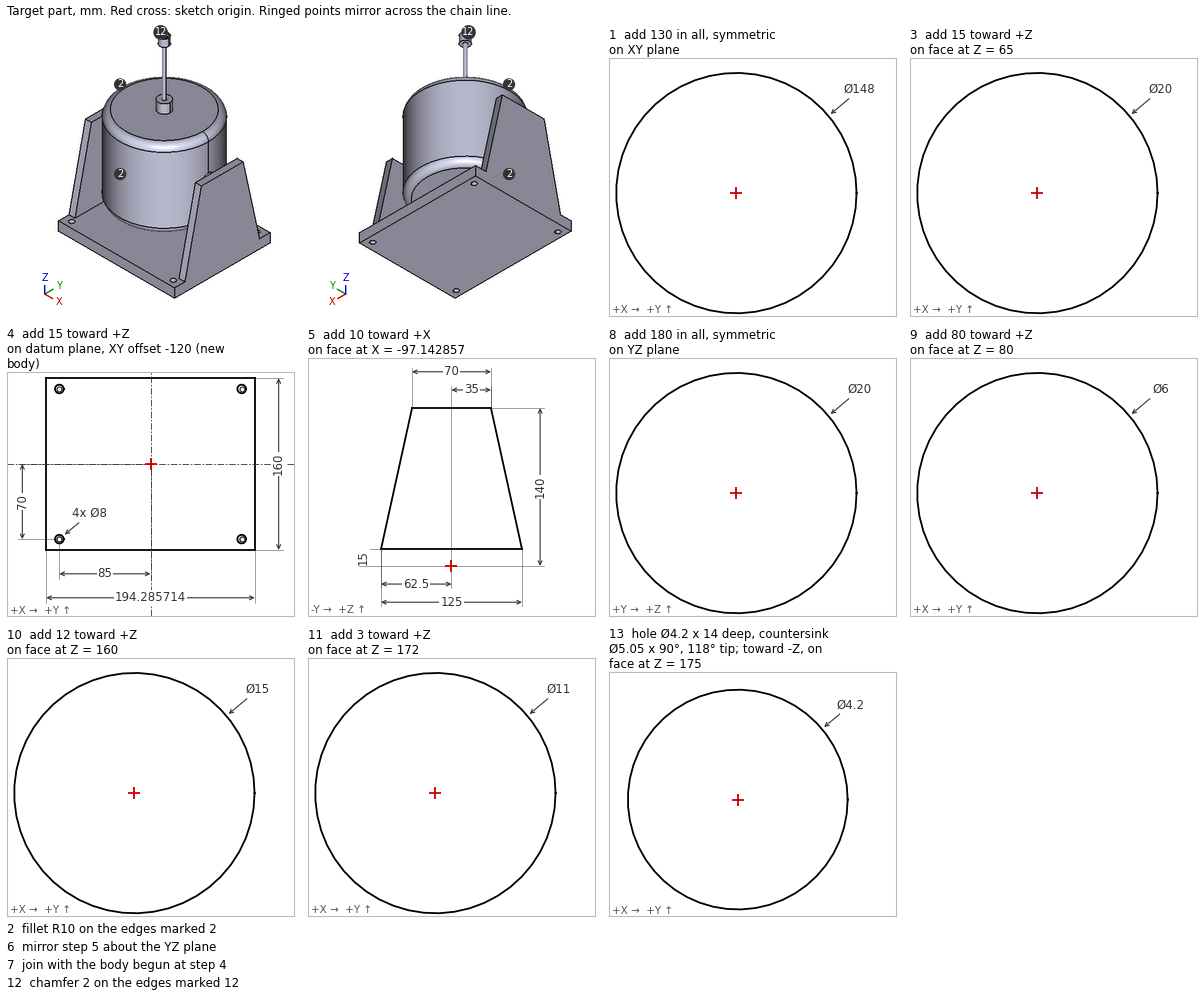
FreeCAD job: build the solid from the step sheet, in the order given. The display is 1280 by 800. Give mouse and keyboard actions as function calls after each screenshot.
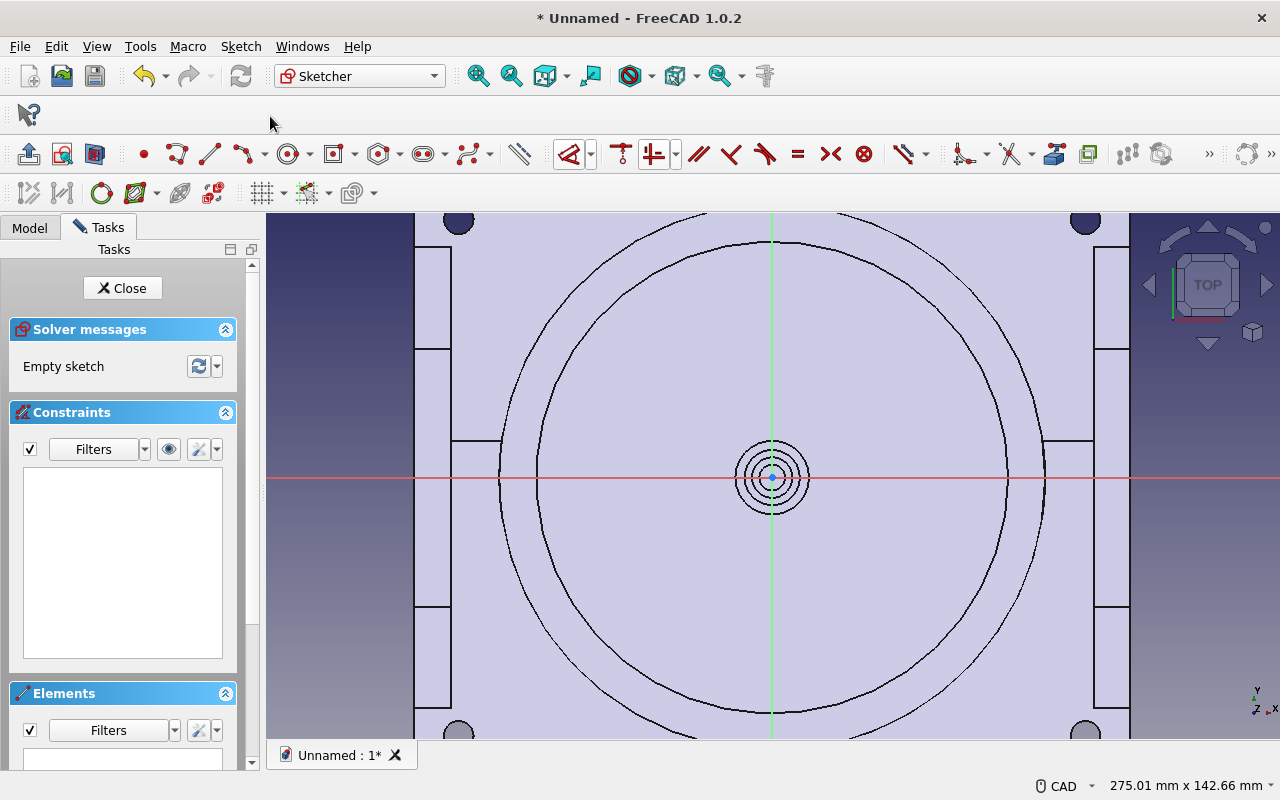
scroll(776, 478, up, 15)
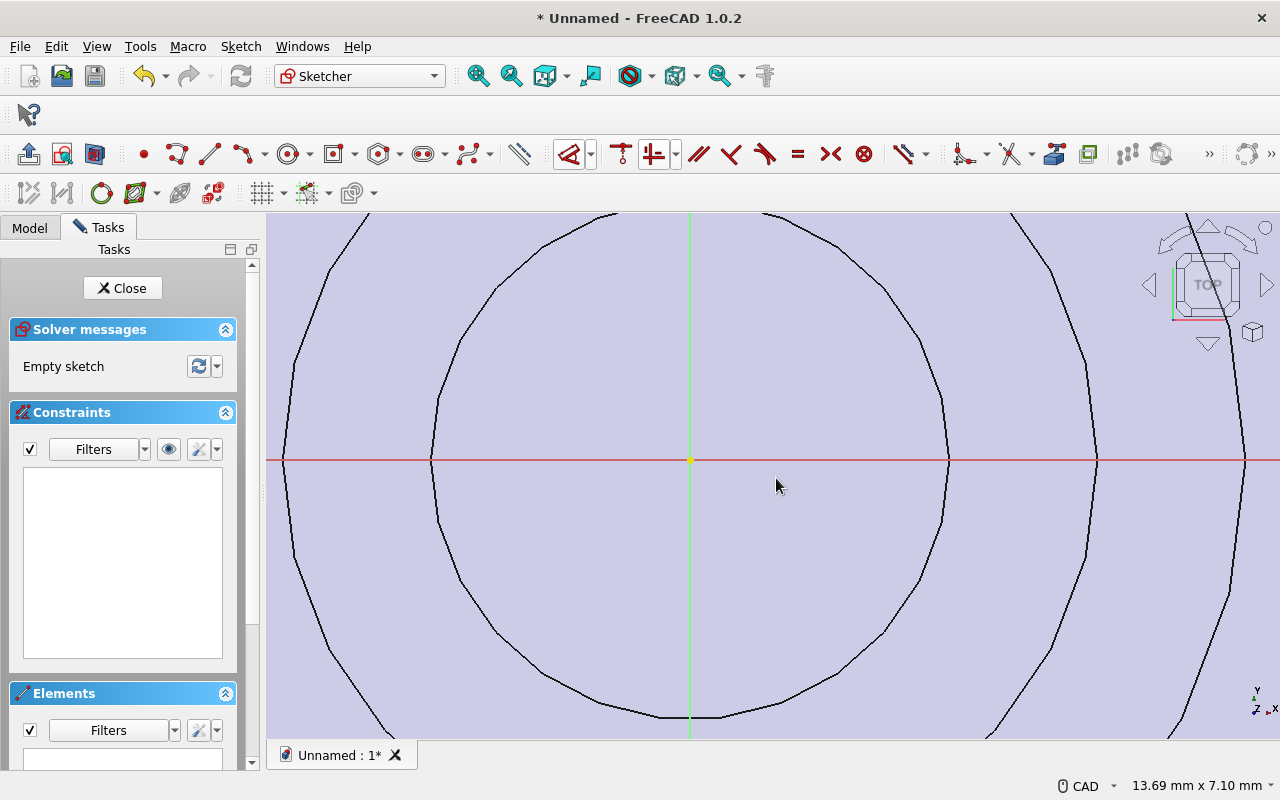
key(g)
key(c)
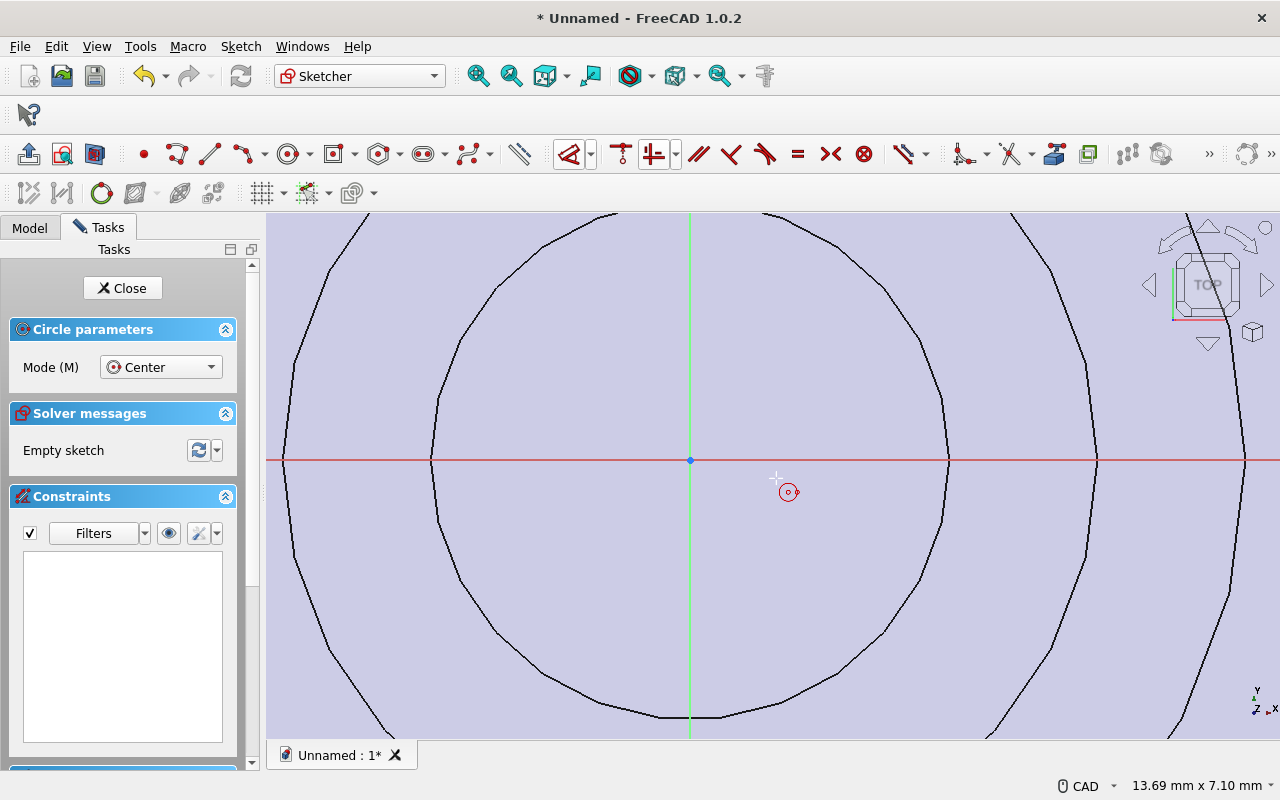
click(690, 460)
click(800, 350)
key(Escape)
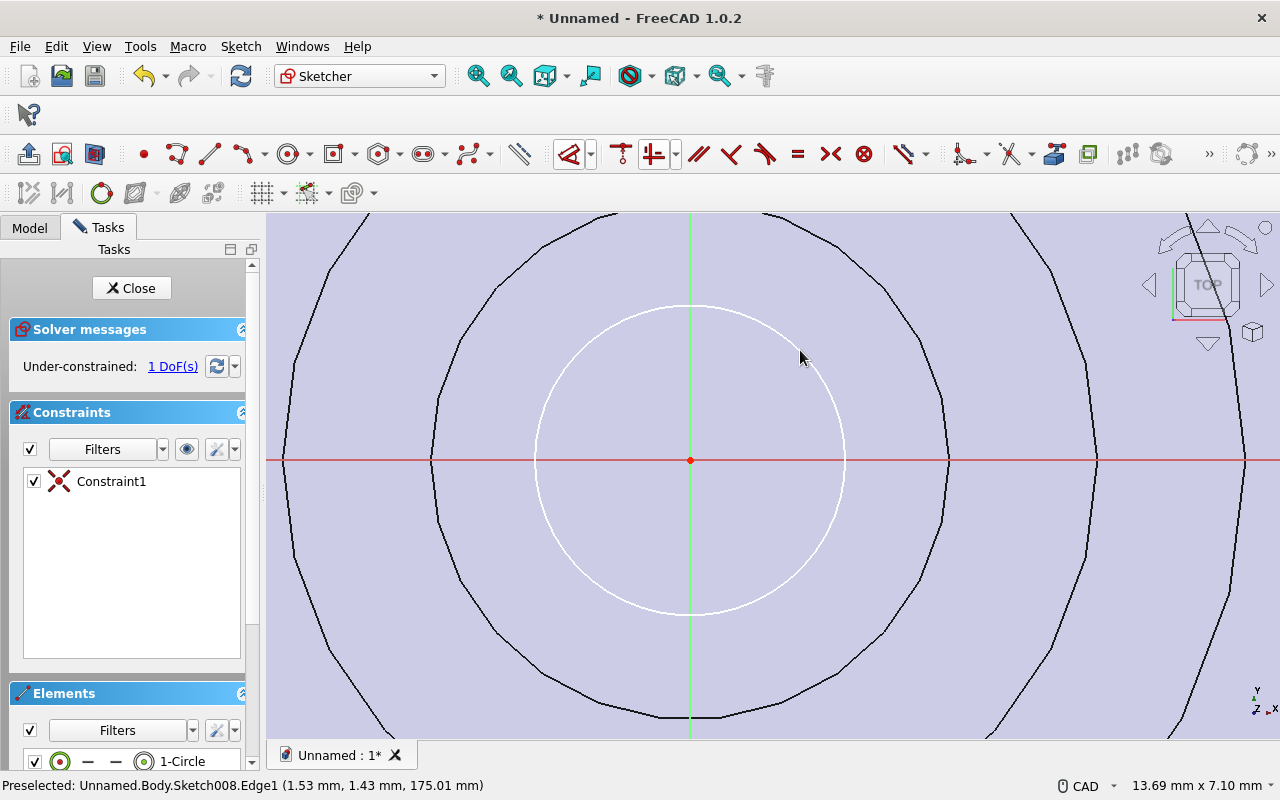
click(799, 350)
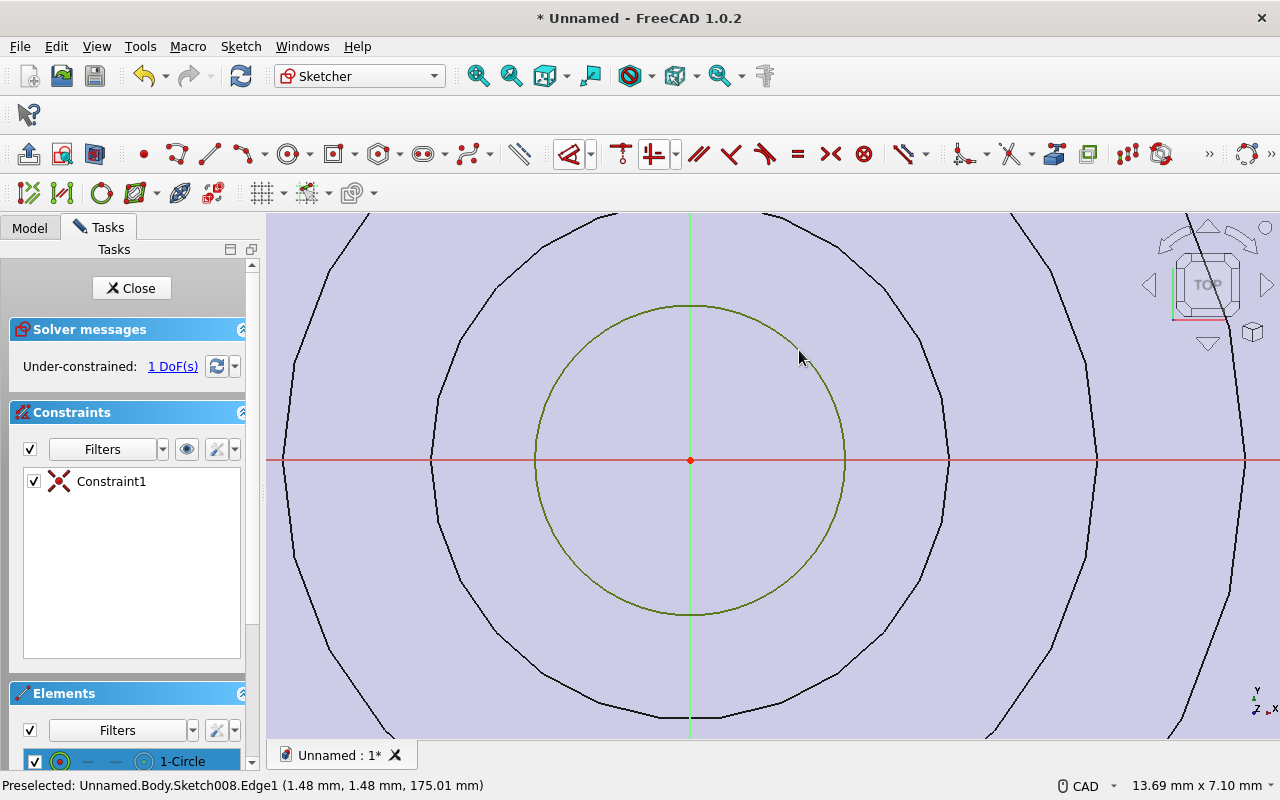
key(k)
key(o)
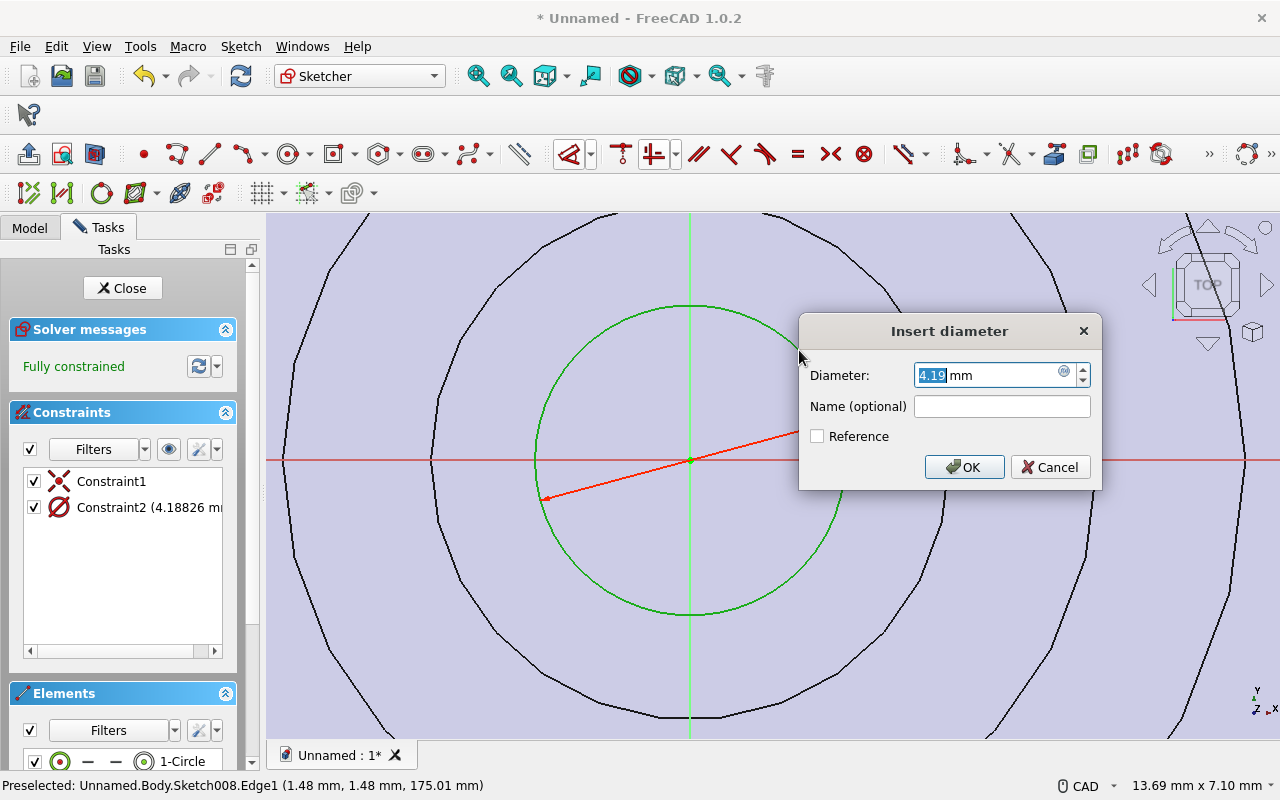
text(4.2)
key(Return)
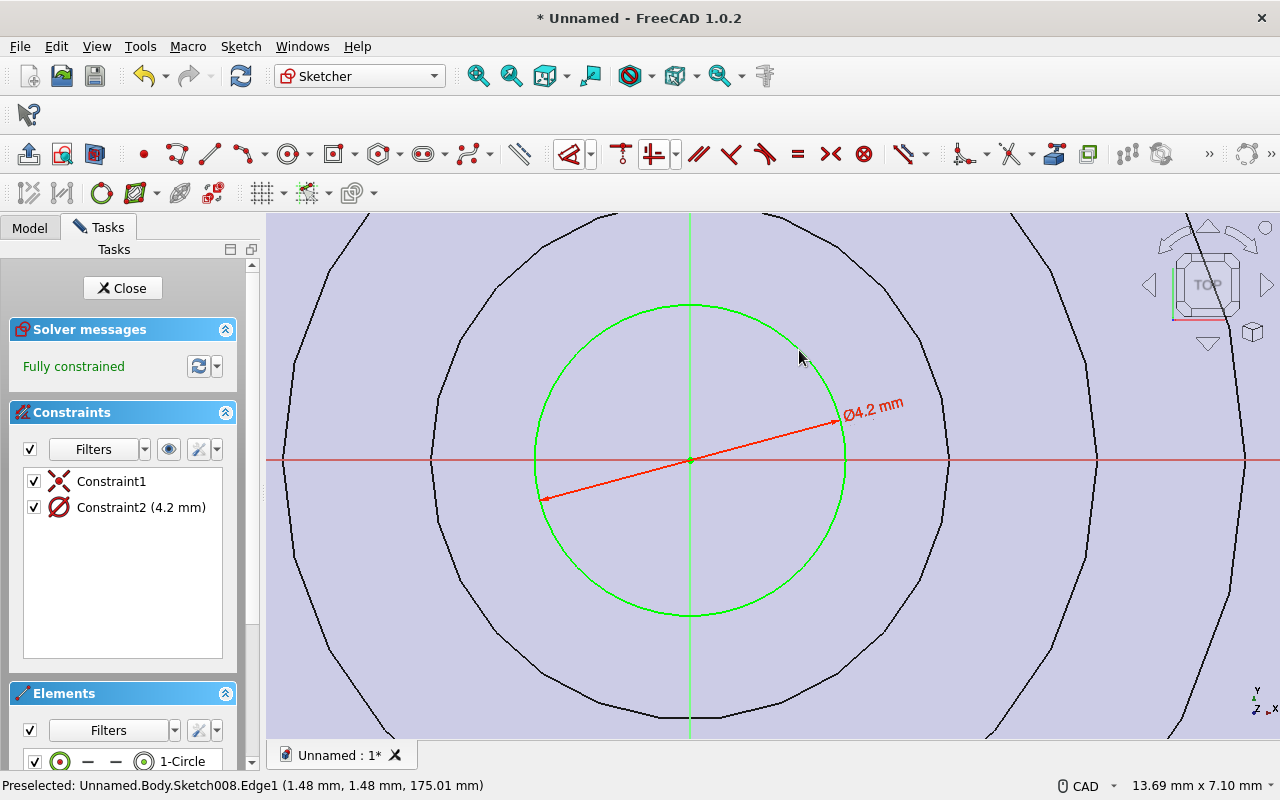
click(123, 288)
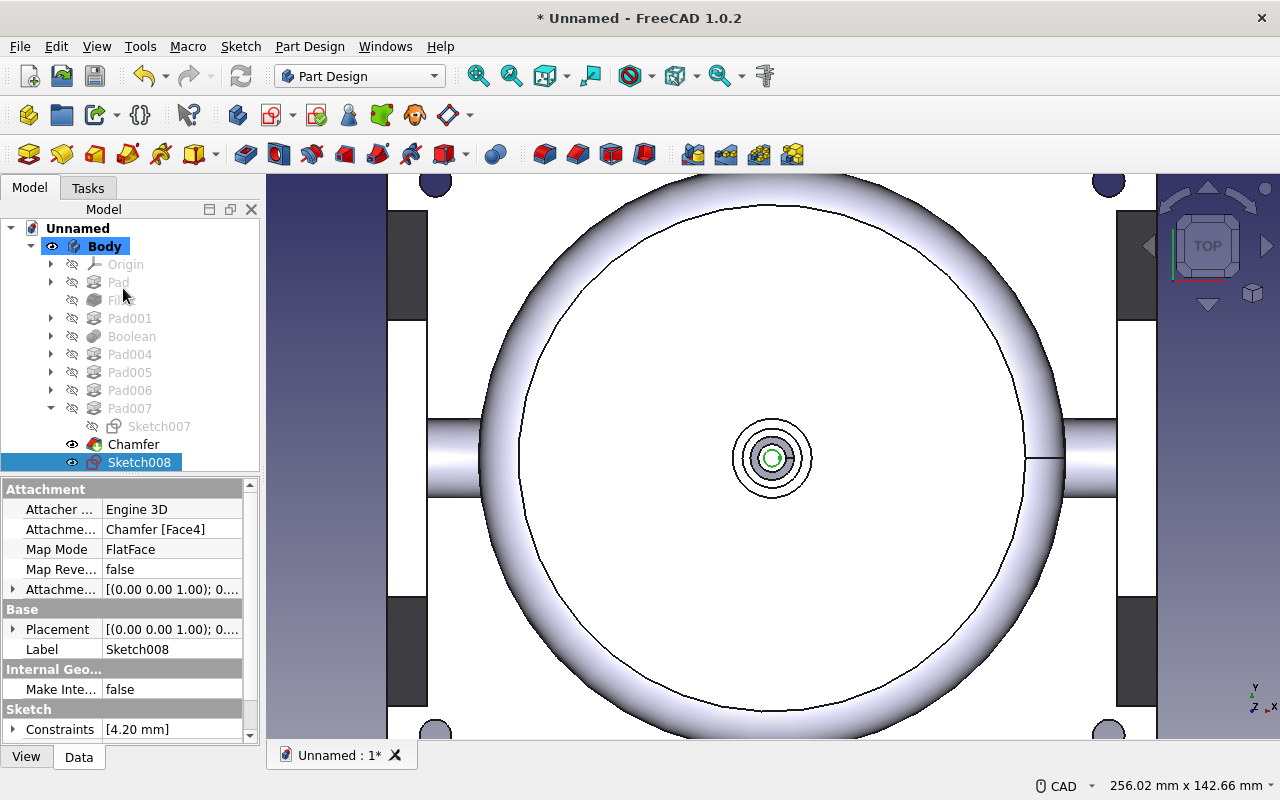
click(279, 154)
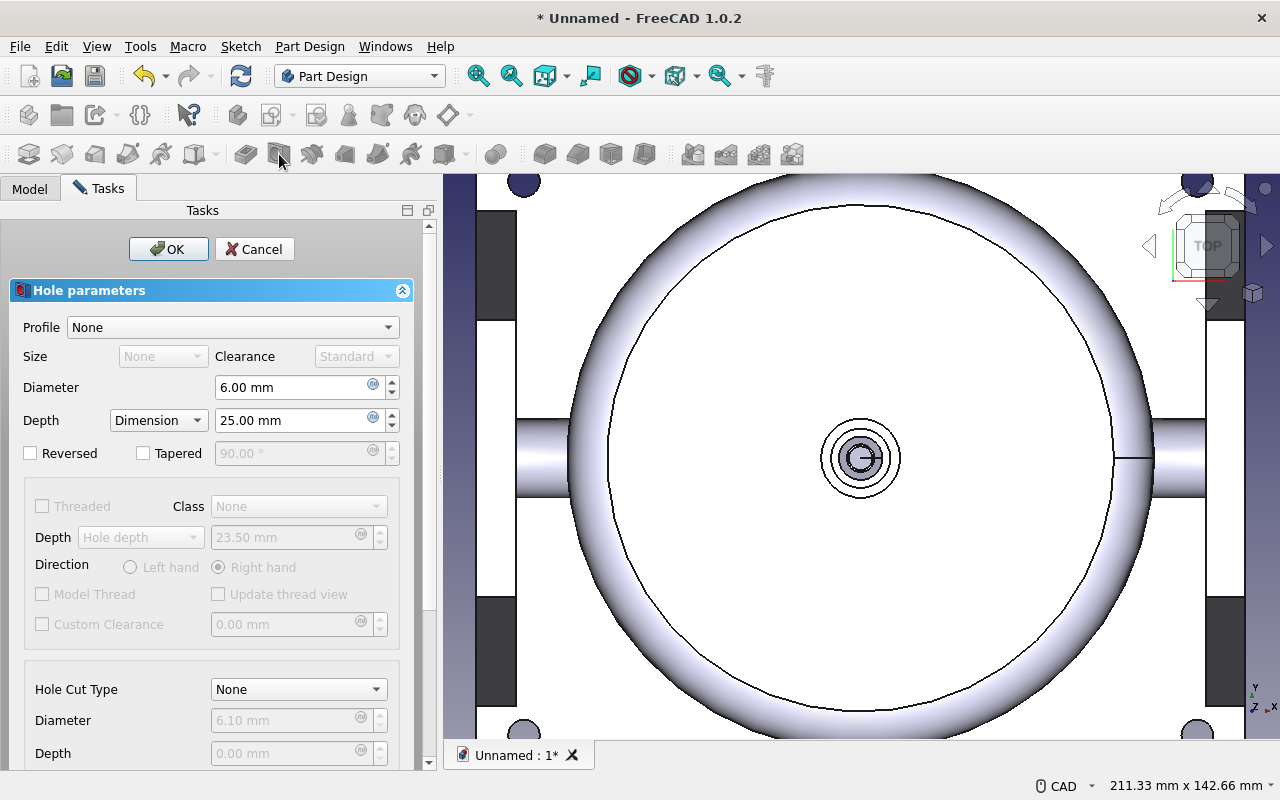
triple_click(300, 388)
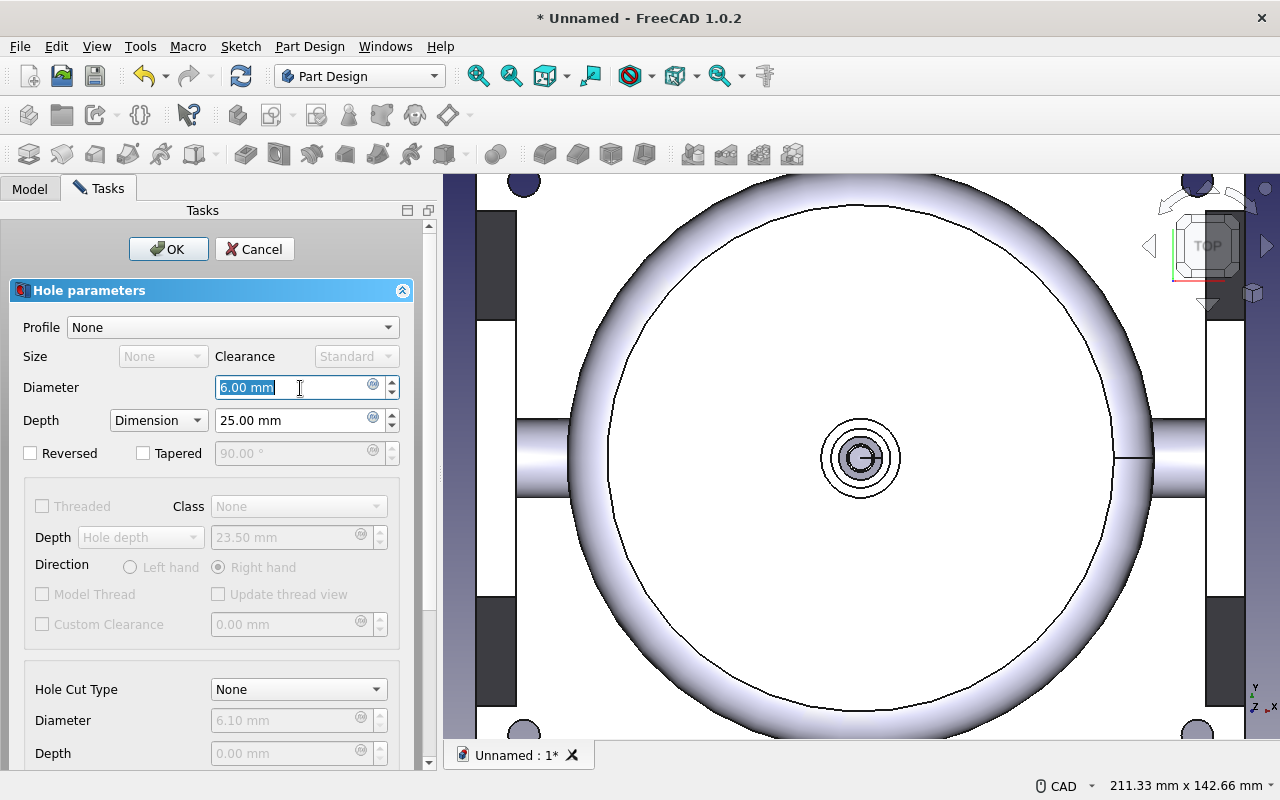
text(4.2)
key(Tab)